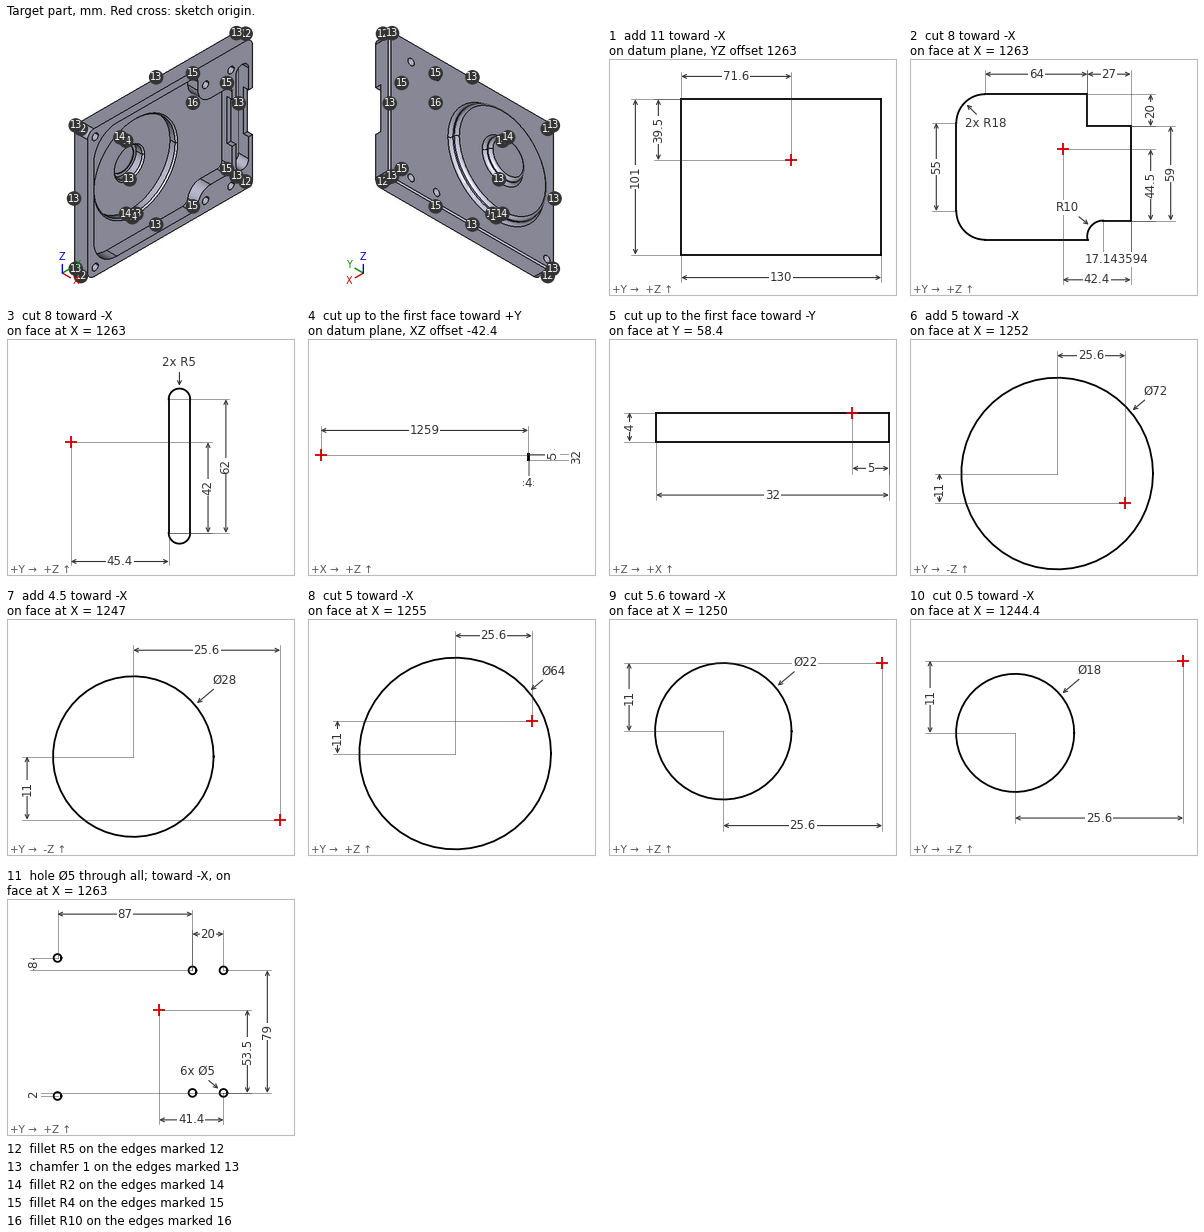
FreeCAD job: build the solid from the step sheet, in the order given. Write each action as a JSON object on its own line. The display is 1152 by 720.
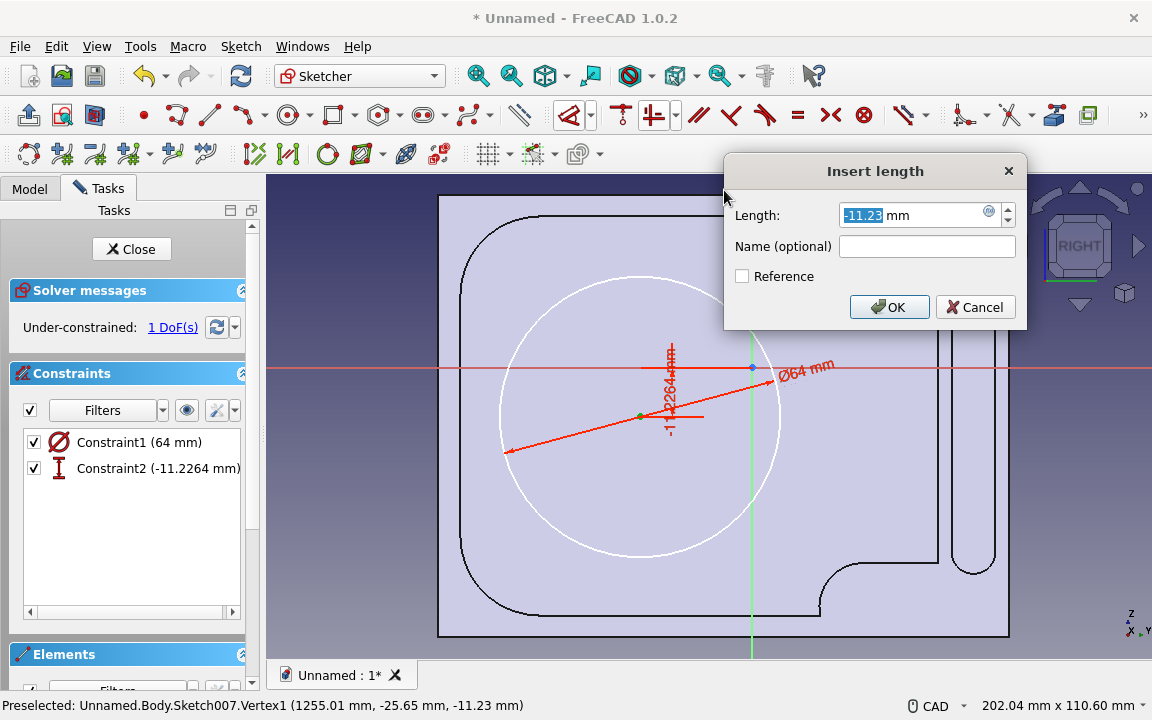
{"action": "type", "text": "-11"}
{"action": "key", "text": "Return"}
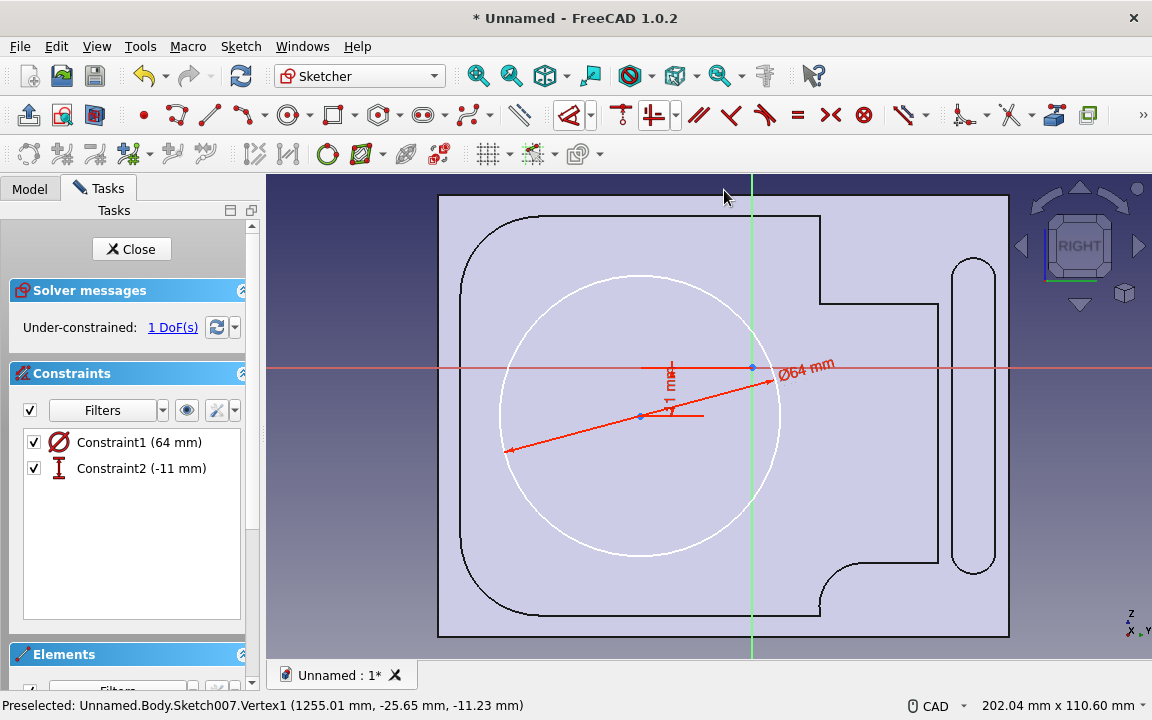
{"action": "left_click", "coordinate": [640, 416]}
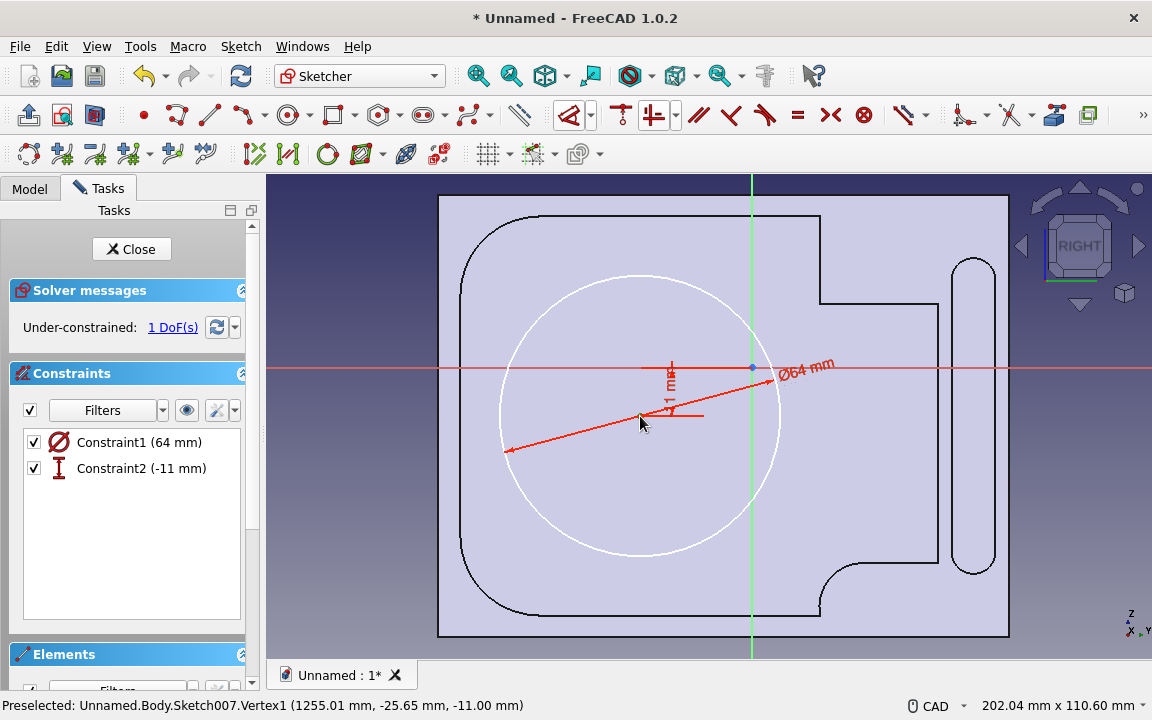
{"action": "left_click", "coordinate": [590, 116]}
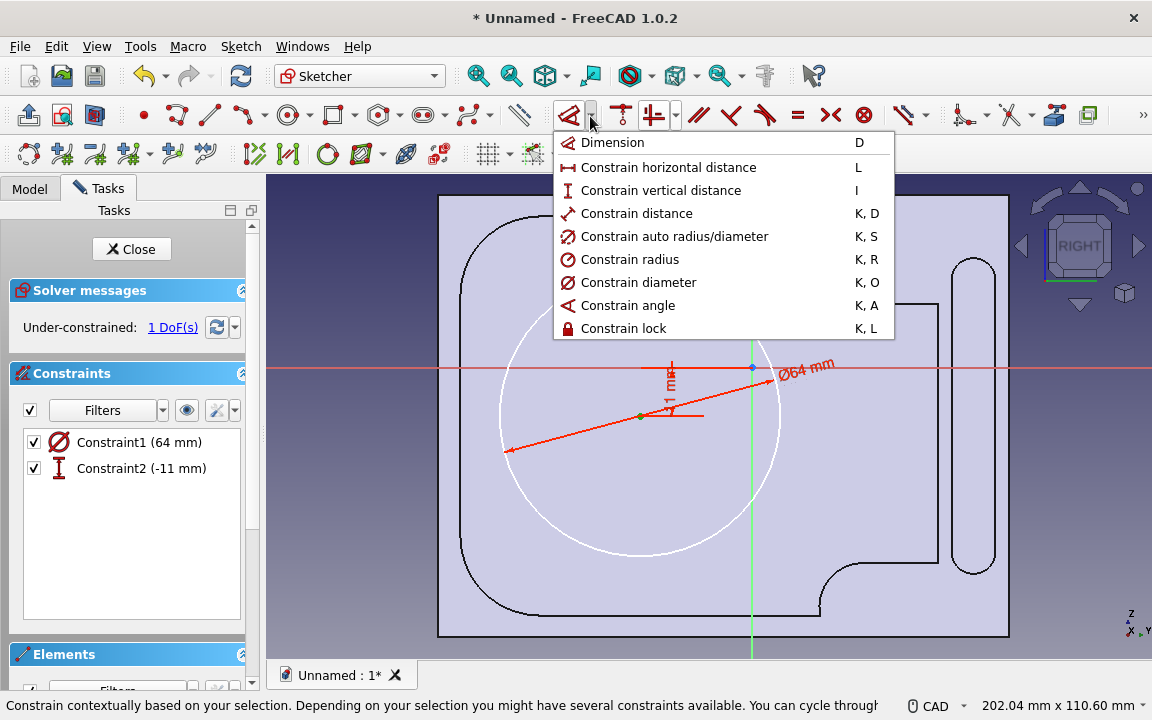
{"action": "left_click", "coordinate": [724, 168]}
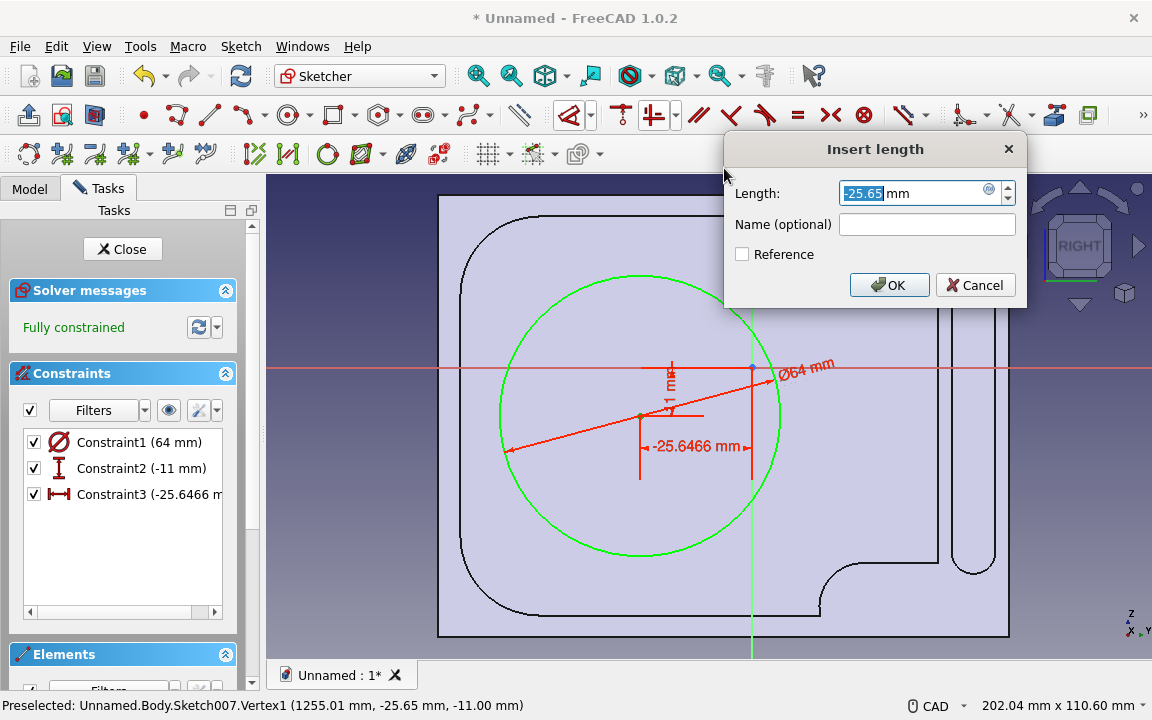
{"action": "type", "text": "-25.6"}
{"action": "key", "text": "Return"}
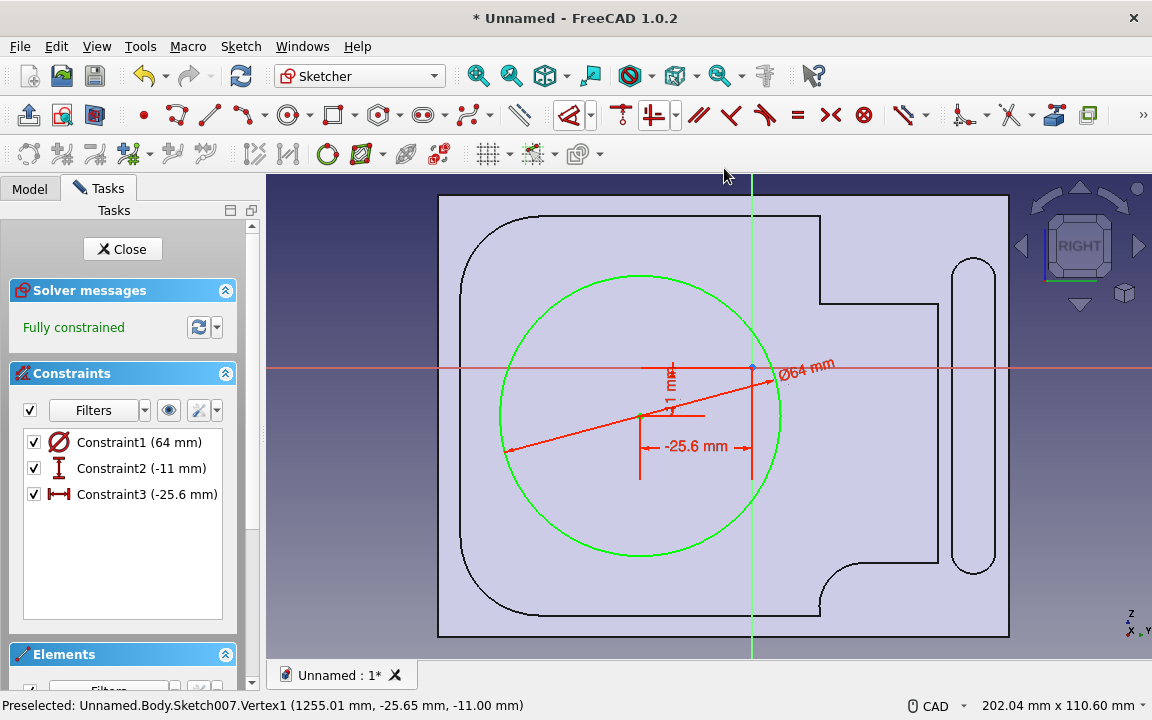
{"action": "left_click", "coordinate": [123, 249]}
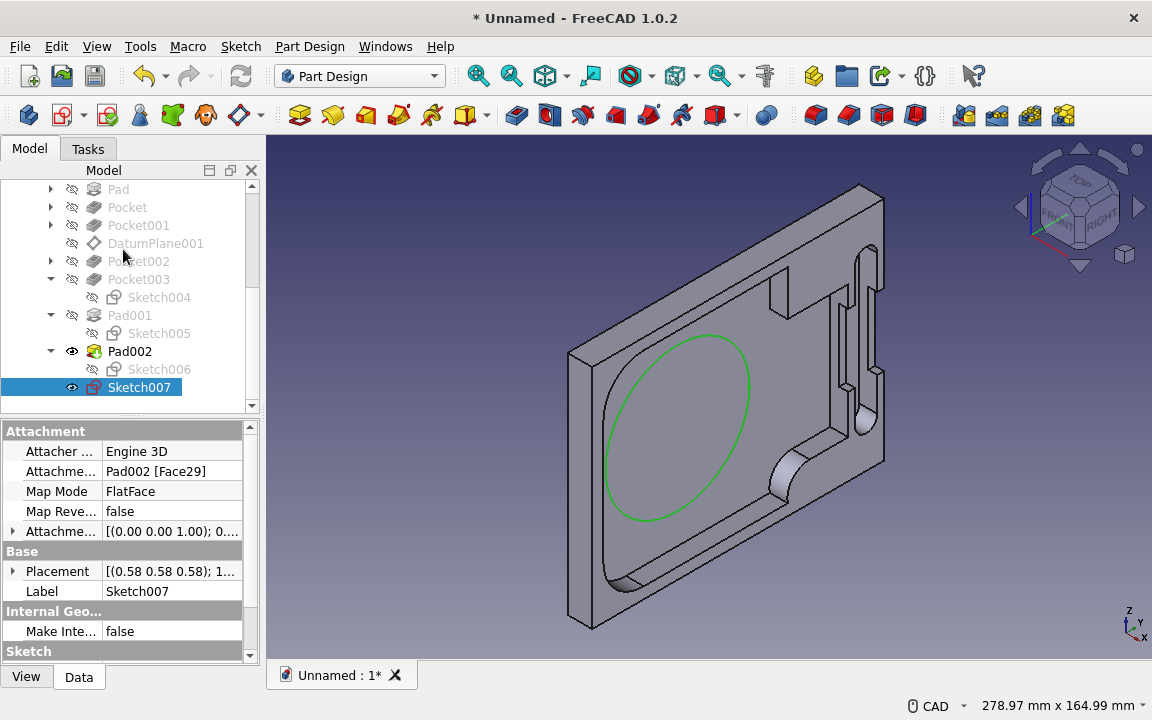
{"action": "left_click", "coordinate": [517, 116]}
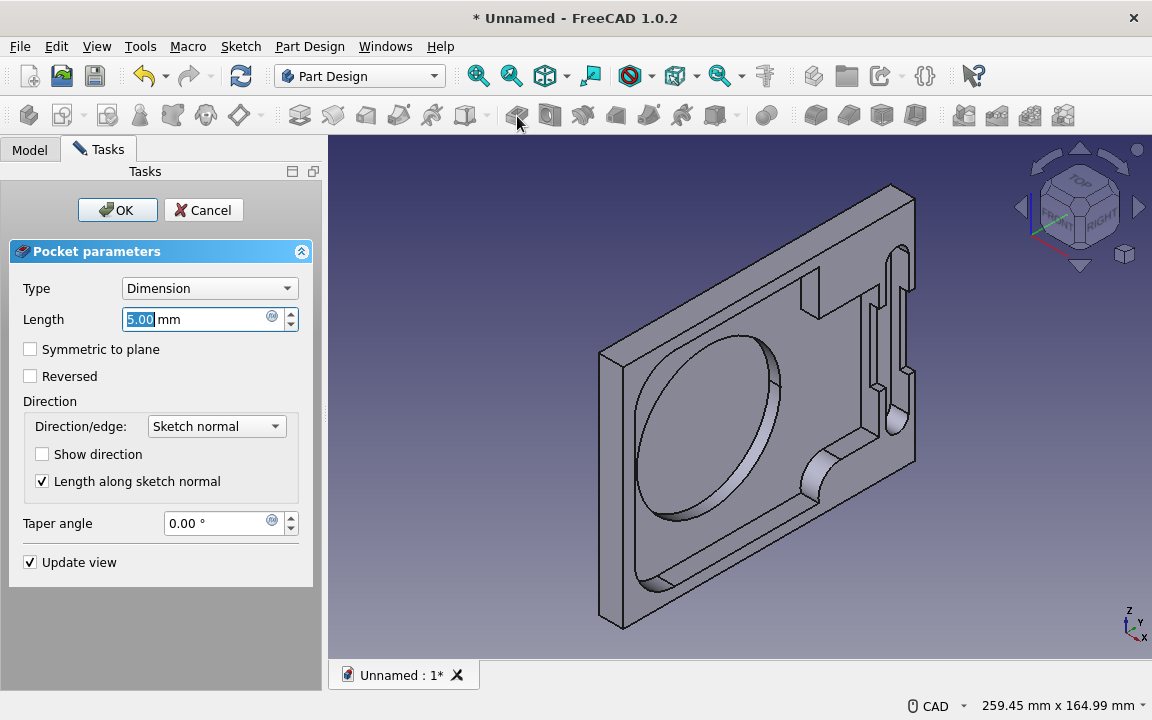
{"action": "type", "text": "5"}
{"action": "key", "text": "Tab"}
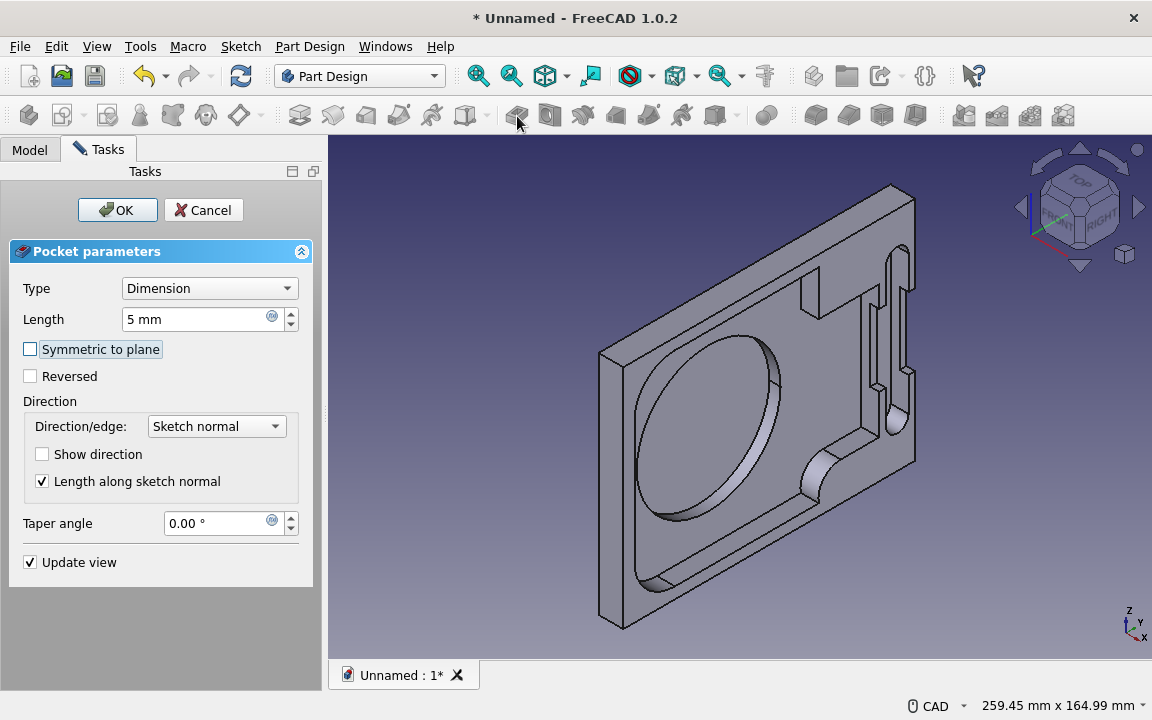
{"action": "left_click", "coordinate": [118, 210]}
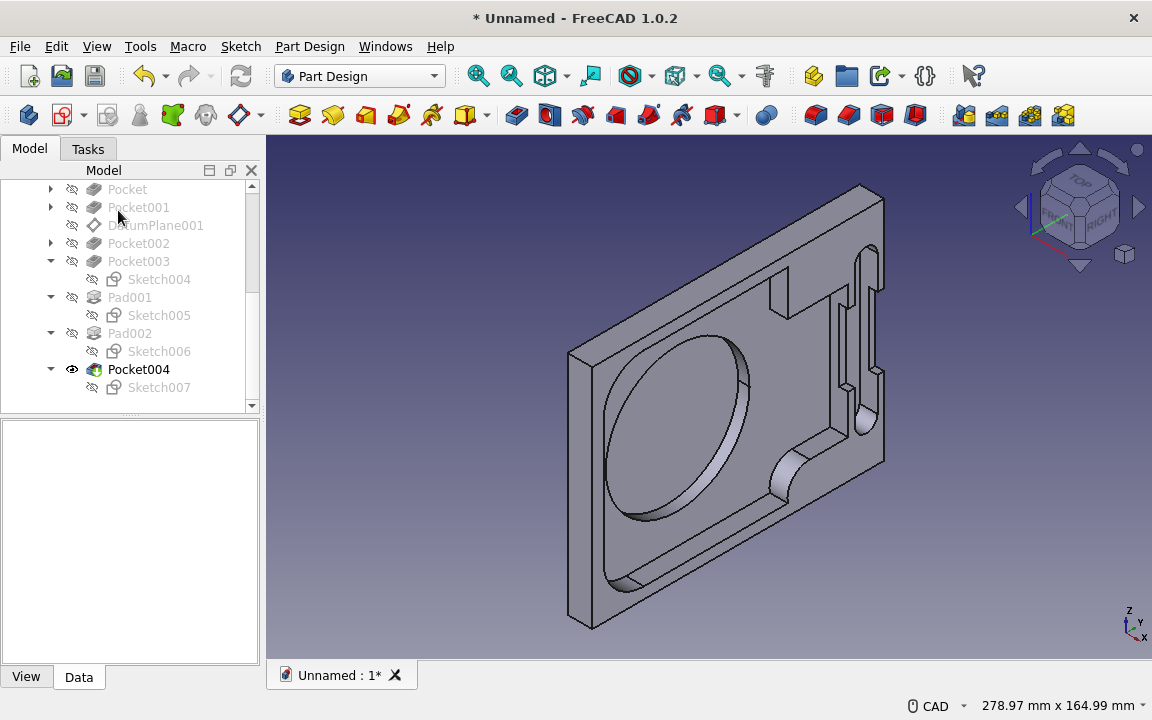
{"action": "left_click", "coordinate": [666, 421]}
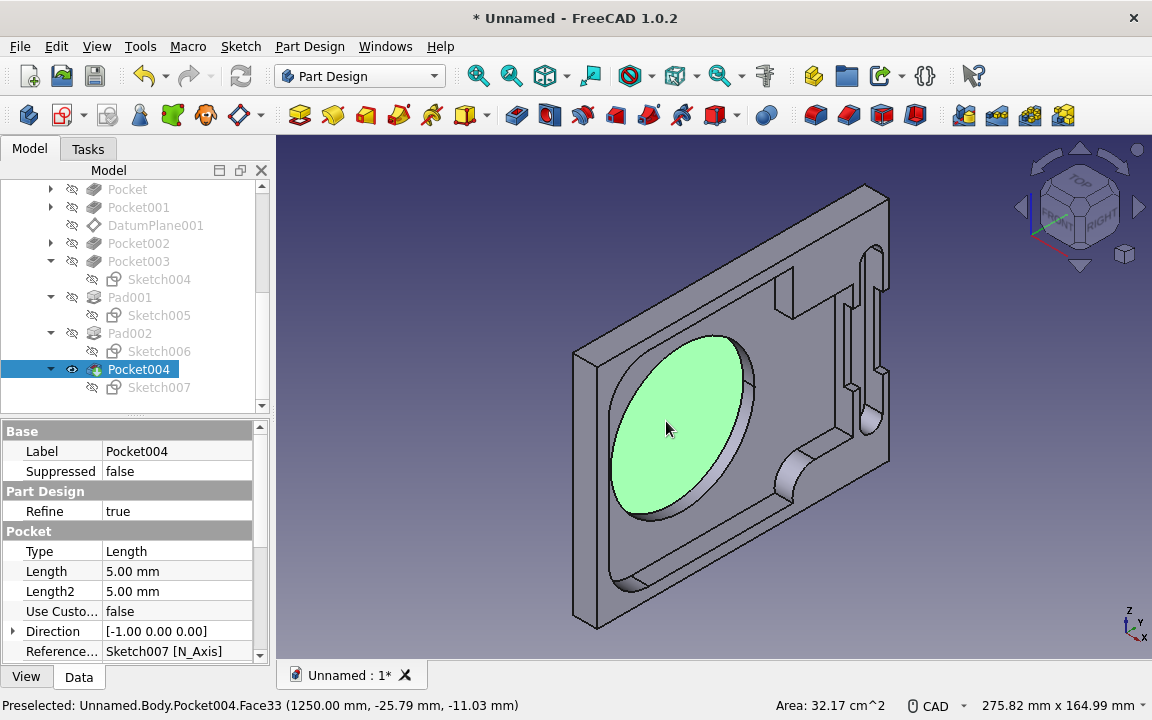
{"action": "left_click", "coordinate": [62, 116]}